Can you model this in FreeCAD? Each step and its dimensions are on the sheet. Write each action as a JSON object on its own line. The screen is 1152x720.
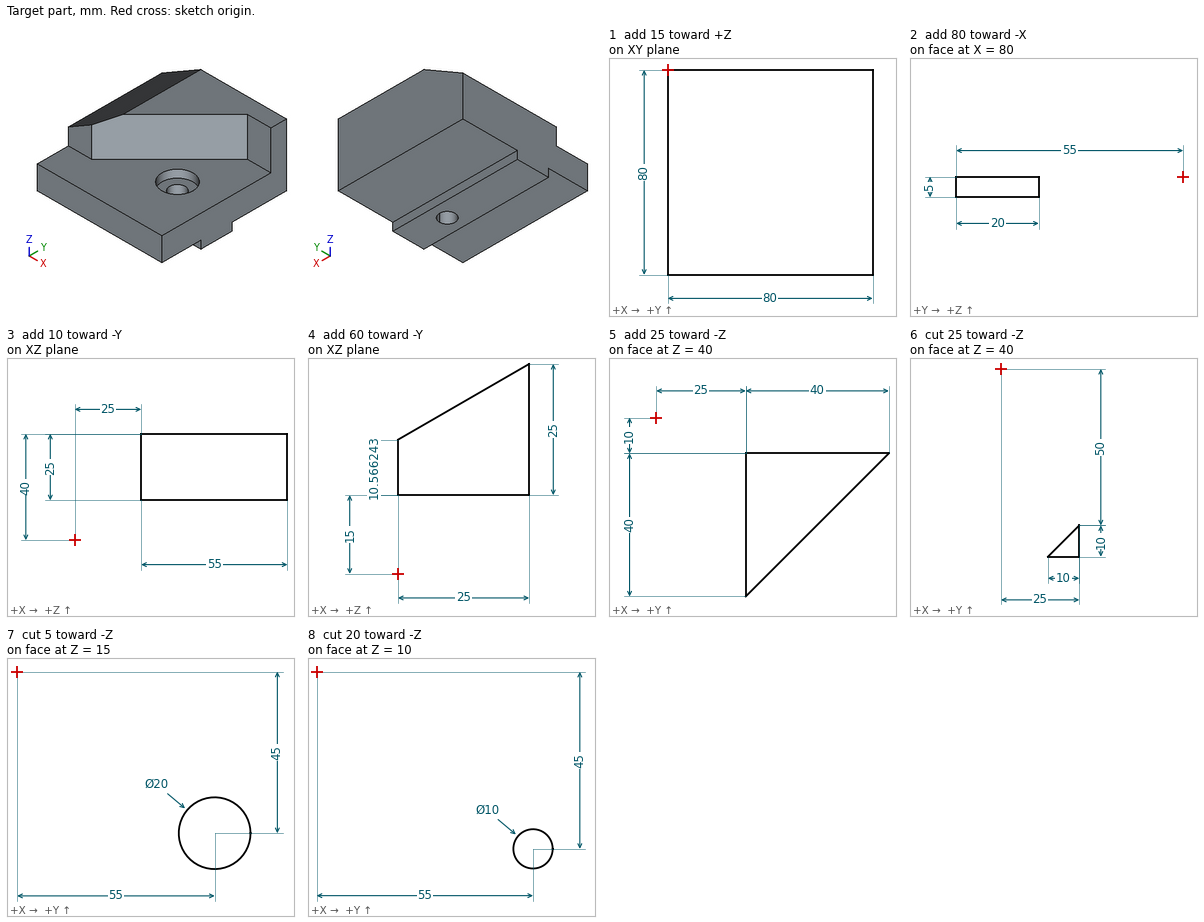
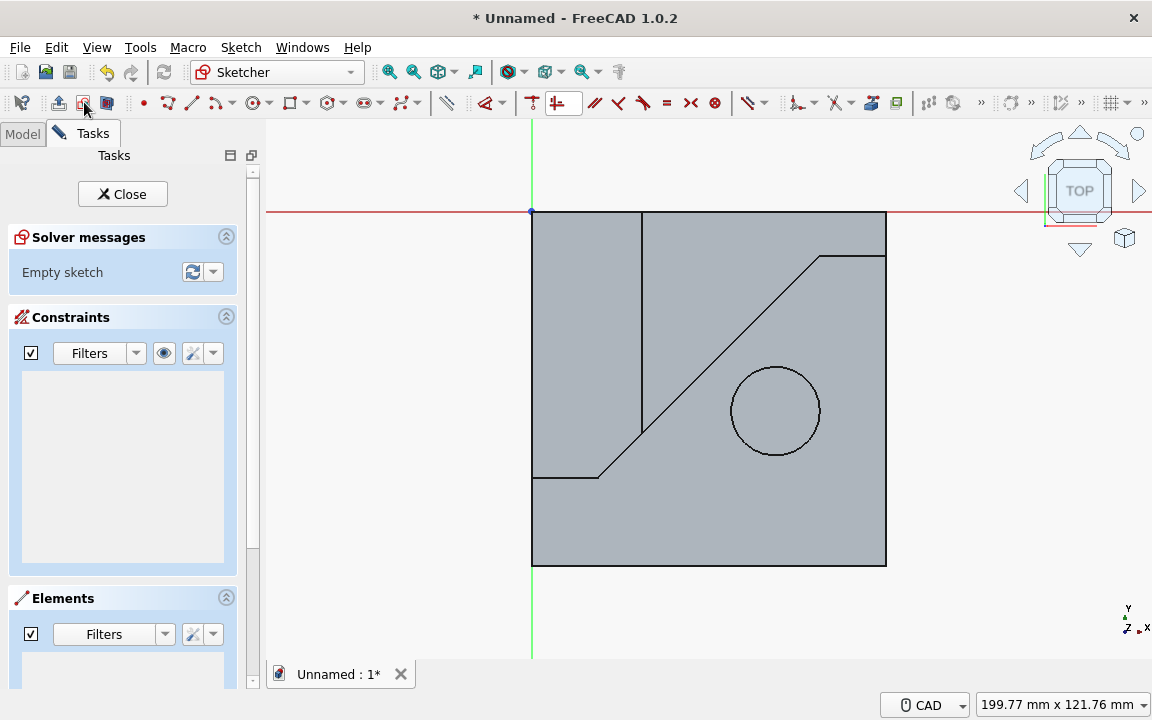
{"action": "left_click", "coordinate": [108, 104]}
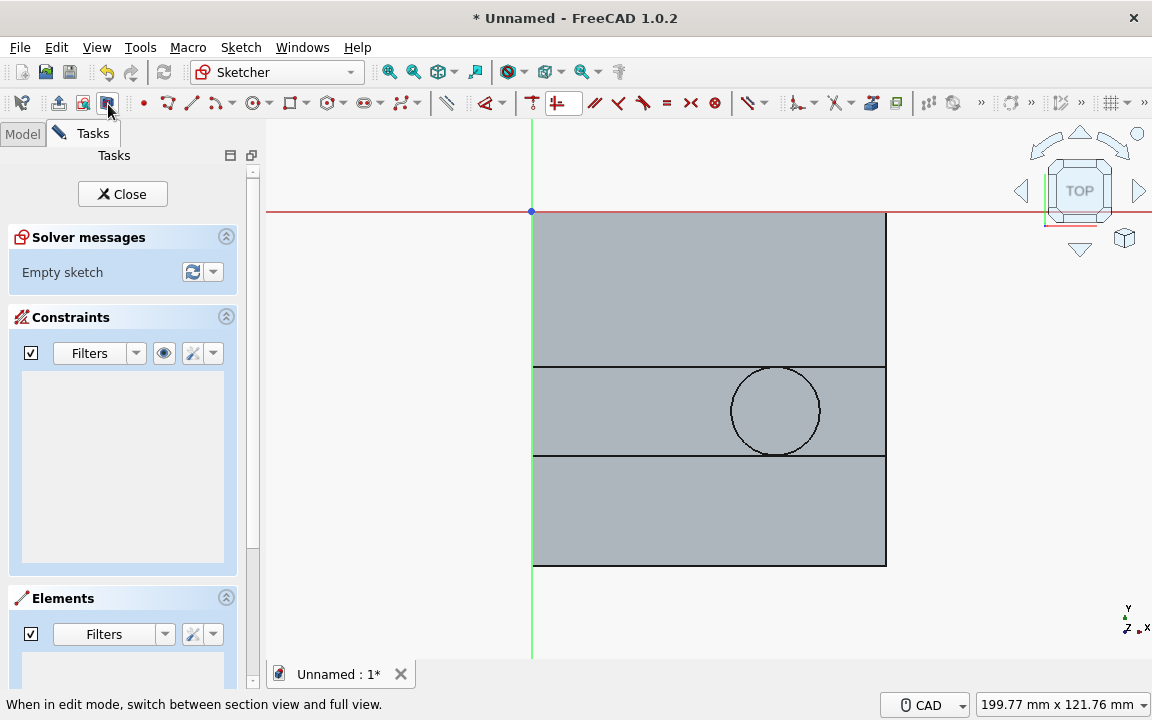
{"action": "scroll", "coordinate": [797, 415], "scroll_direction": "up", "scroll_amount": 10}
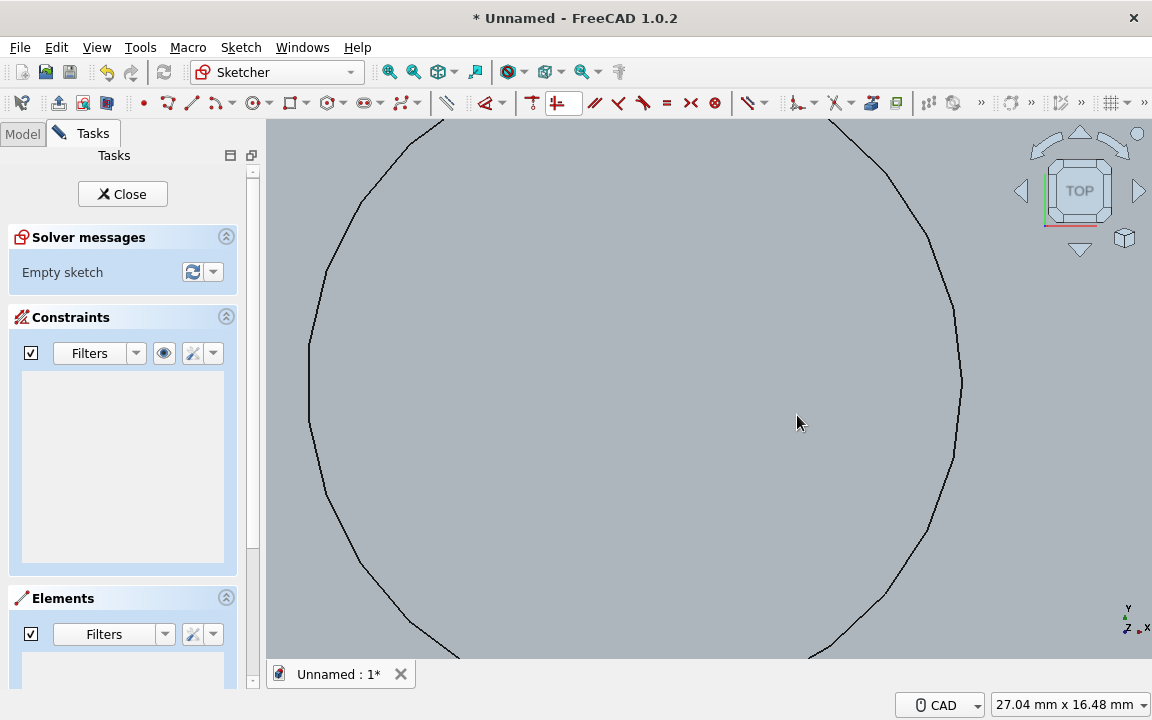
{"action": "left_click", "coordinate": [254, 104]}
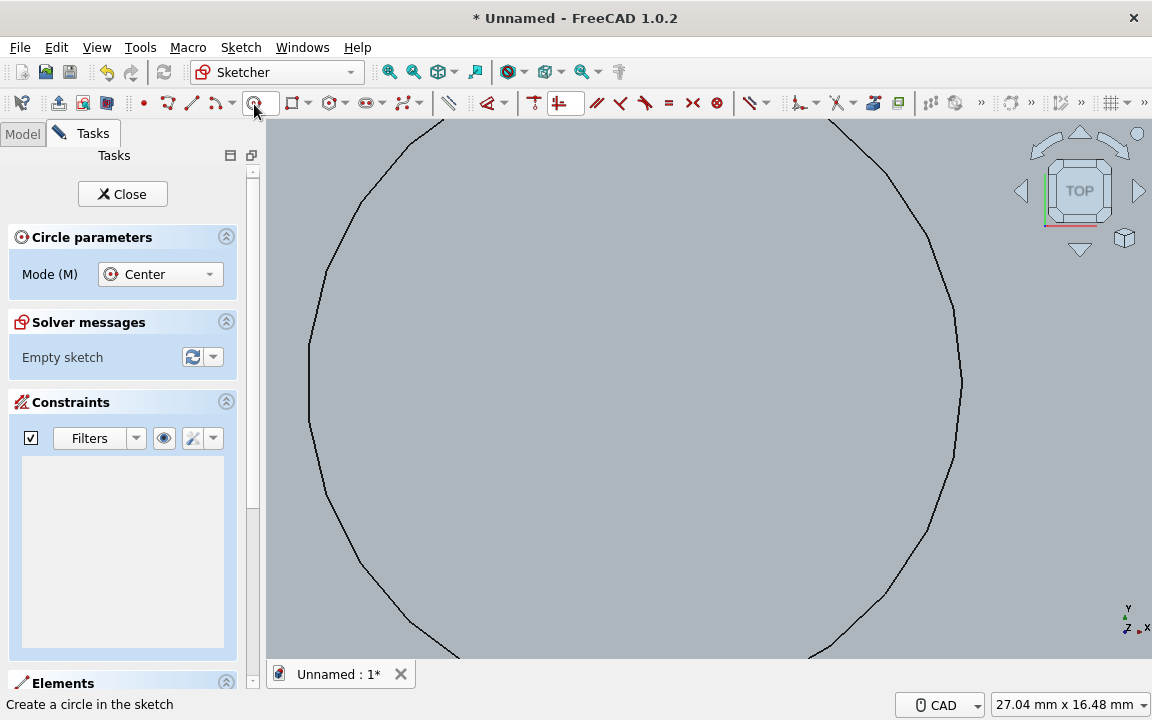
{"action": "left_click", "coordinate": [634, 383]}
{"action": "left_click", "coordinate": [750, 267]}
{"action": "key", "text": "Escape"}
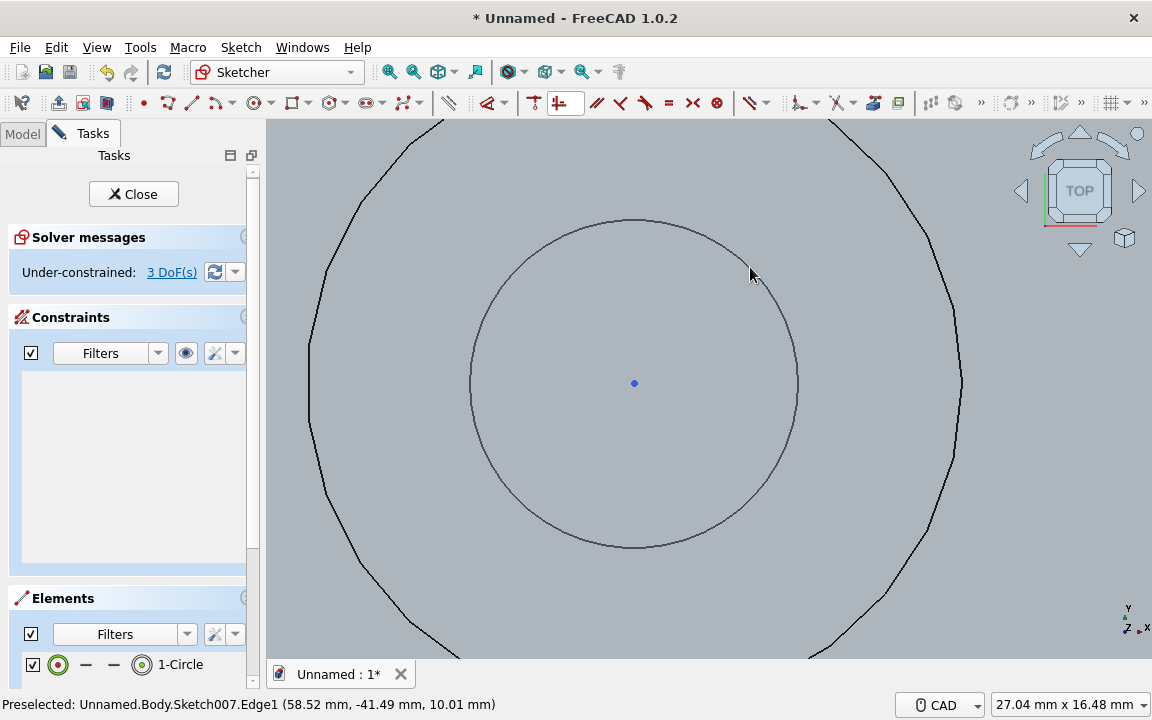
{"action": "left_click", "coordinate": [488, 104]}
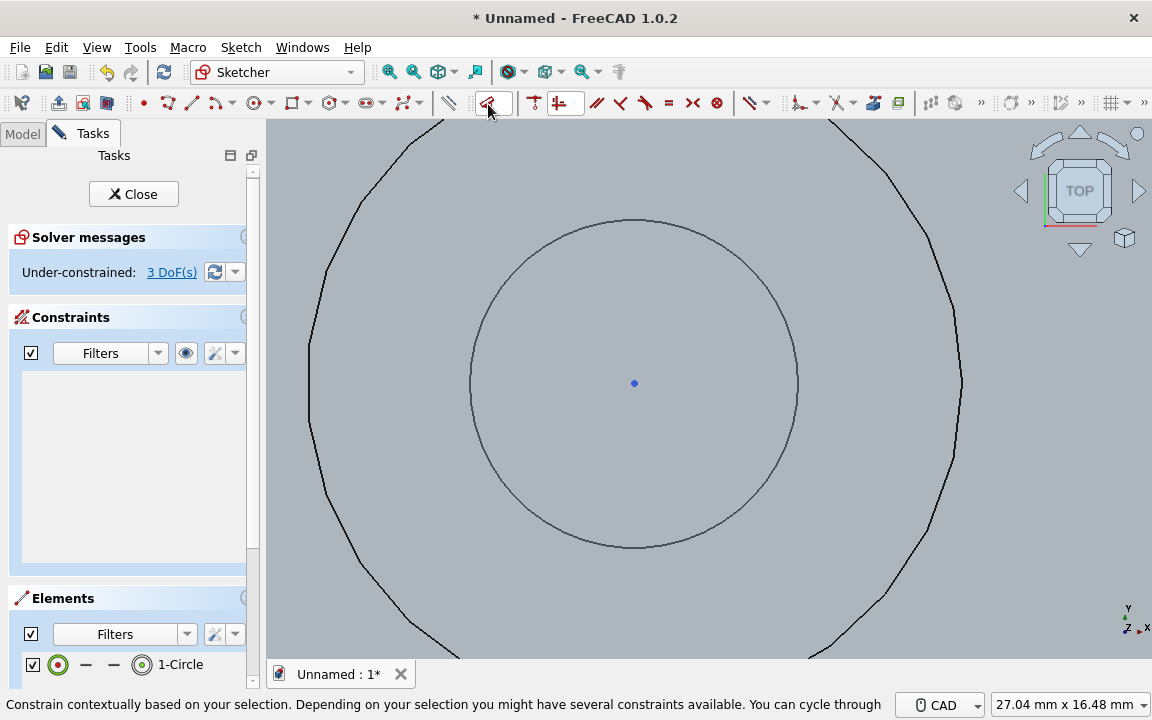
{"action": "left_click", "coordinate": [750, 268]}
{"action": "left_click", "coordinate": [773, 245]}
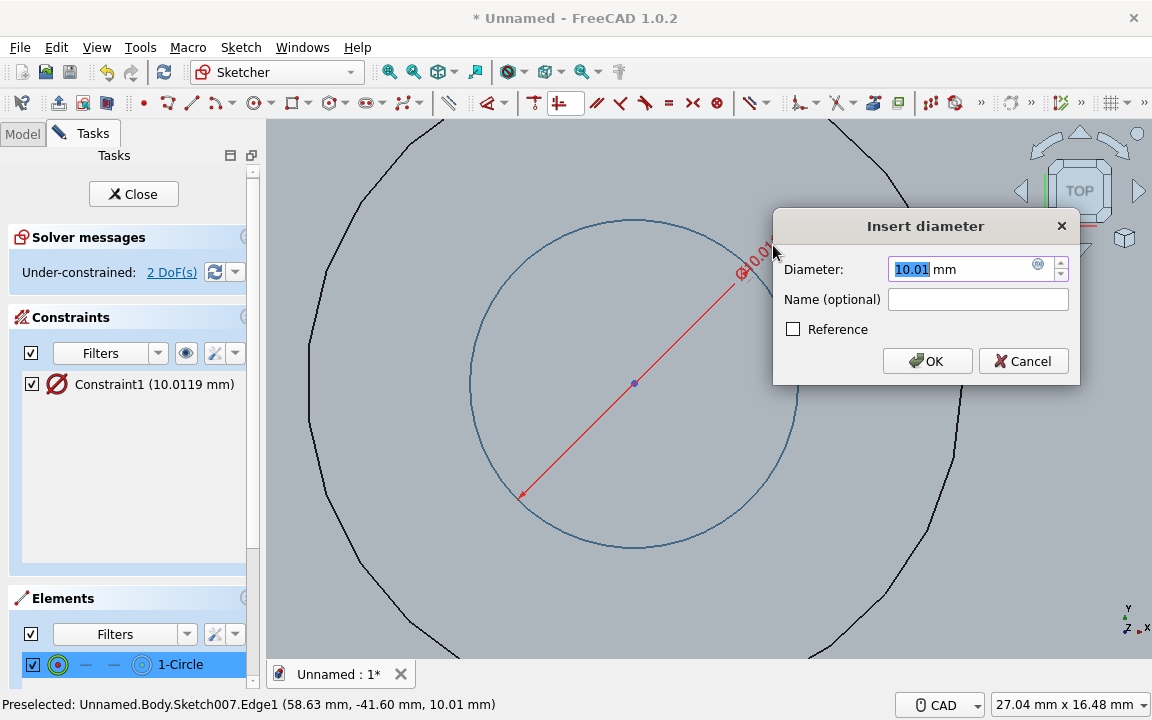
{"action": "type", "text": "10"}
{"action": "key", "text": "Return"}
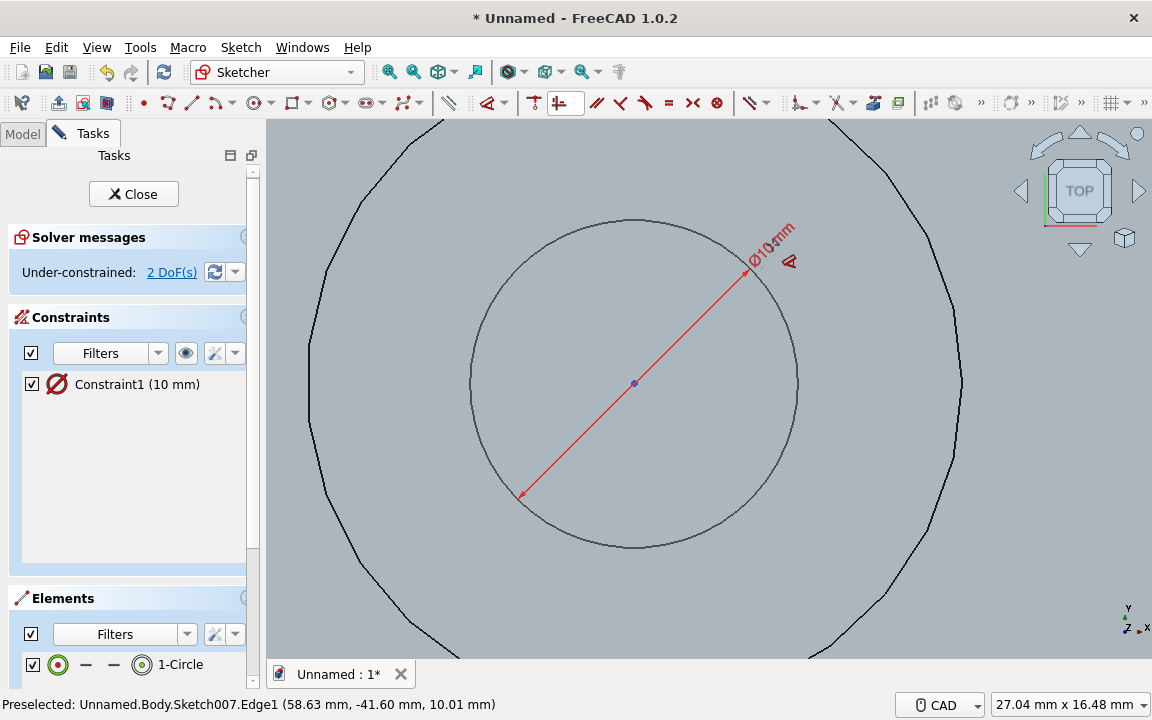
{"action": "left_click", "coordinate": [634, 384]}
{"action": "left_click", "coordinate": [386, 418]}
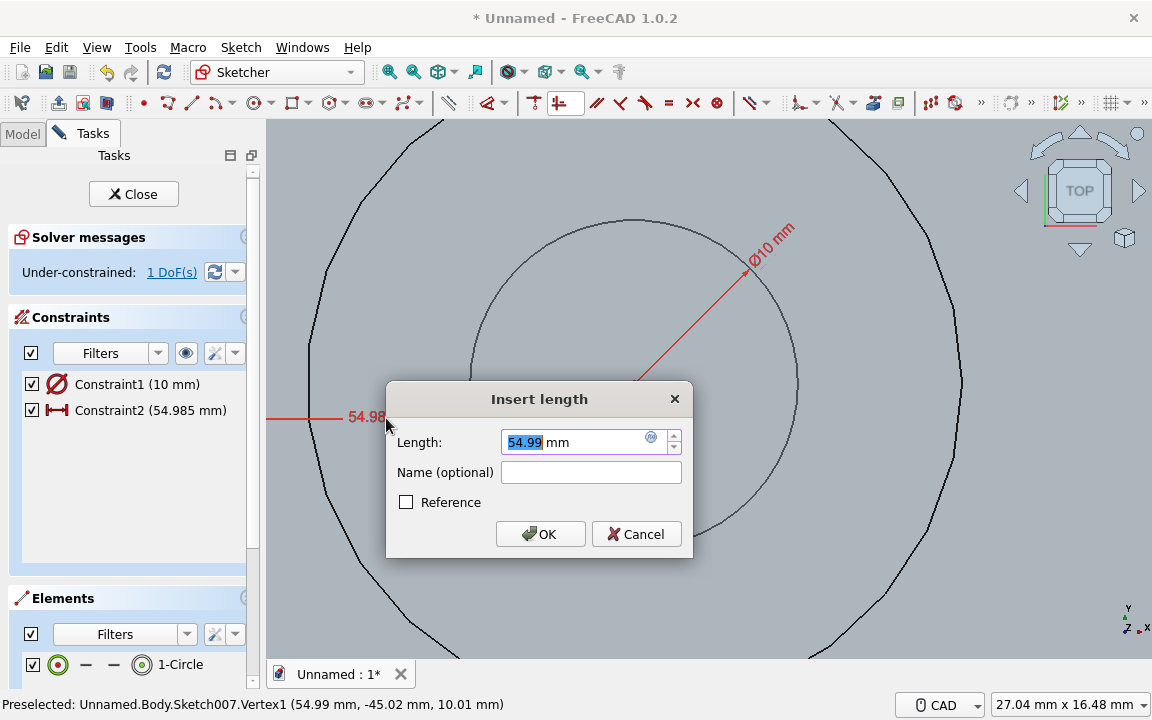
{"action": "type", "text": "55"}
{"action": "key", "text": "Return"}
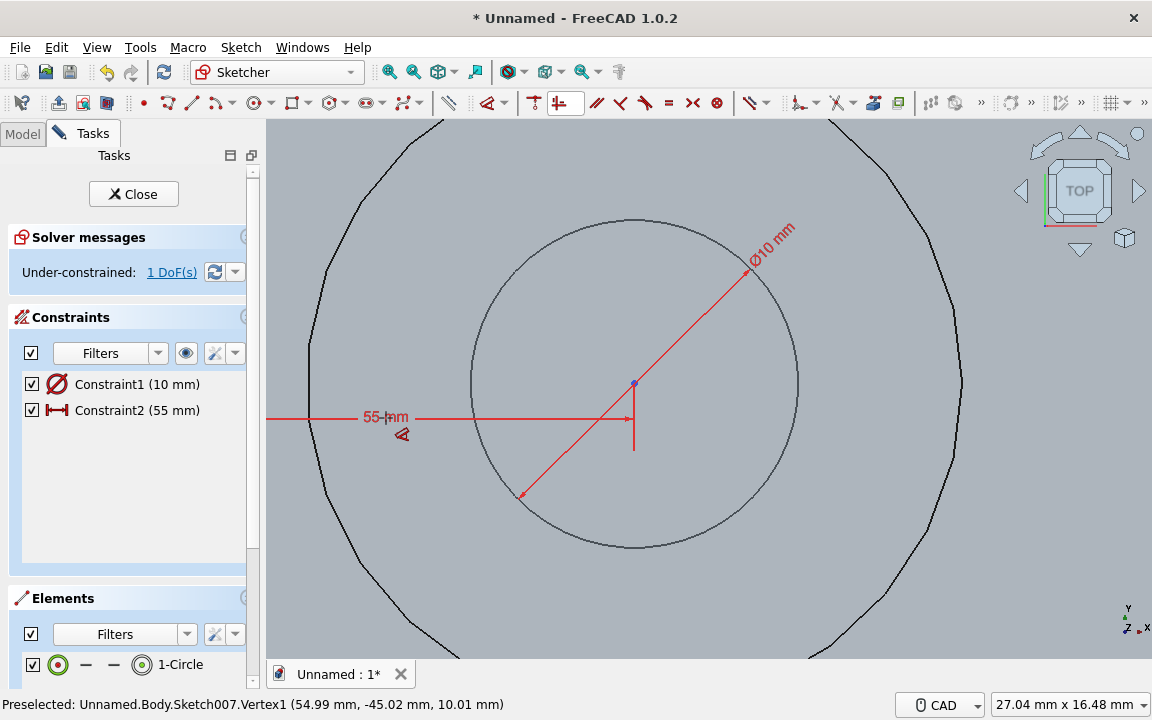
{"action": "left_click", "coordinate": [634, 384]}
{"action": "left_click", "coordinate": [668, 265]}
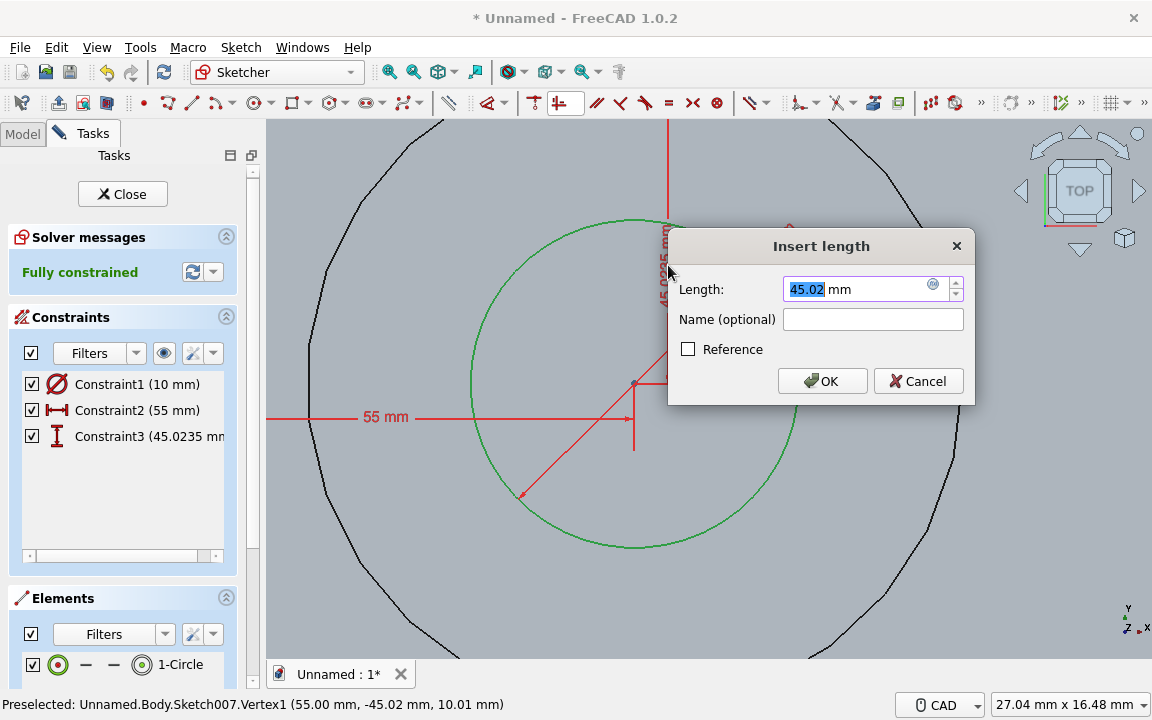
{"action": "type", "text": "45"}
{"action": "key", "text": "Return"}
{"action": "key", "text": "Escape"}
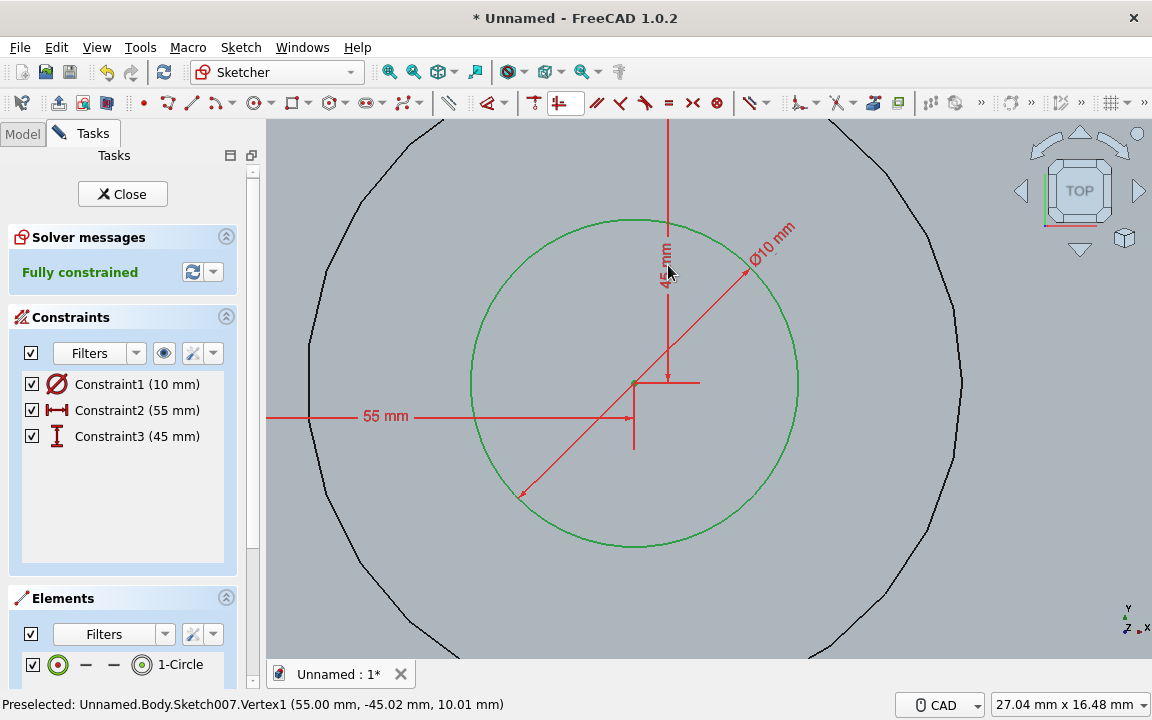
{"action": "left_click", "coordinate": [123, 194]}